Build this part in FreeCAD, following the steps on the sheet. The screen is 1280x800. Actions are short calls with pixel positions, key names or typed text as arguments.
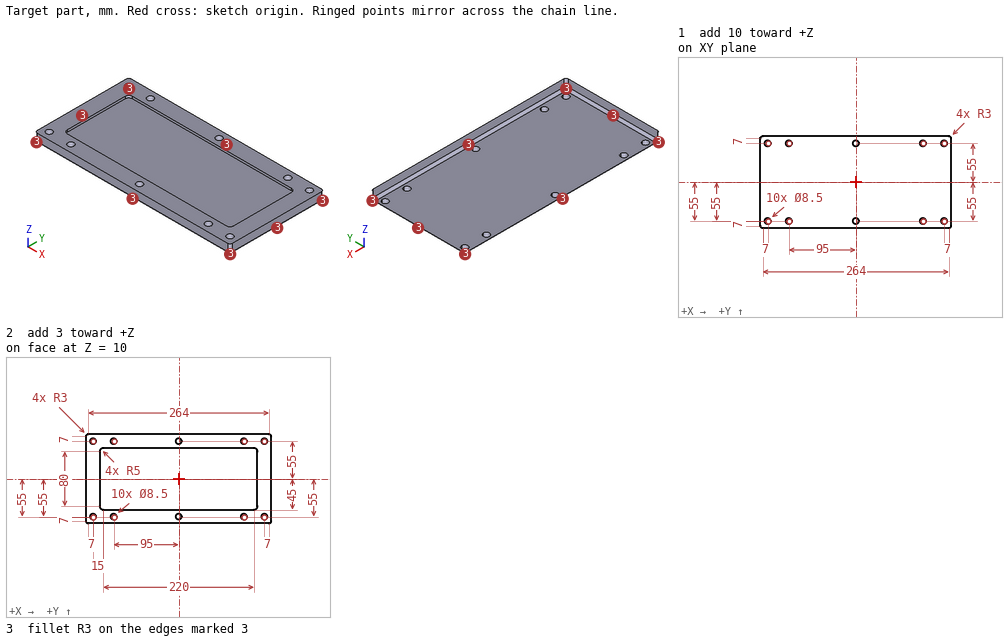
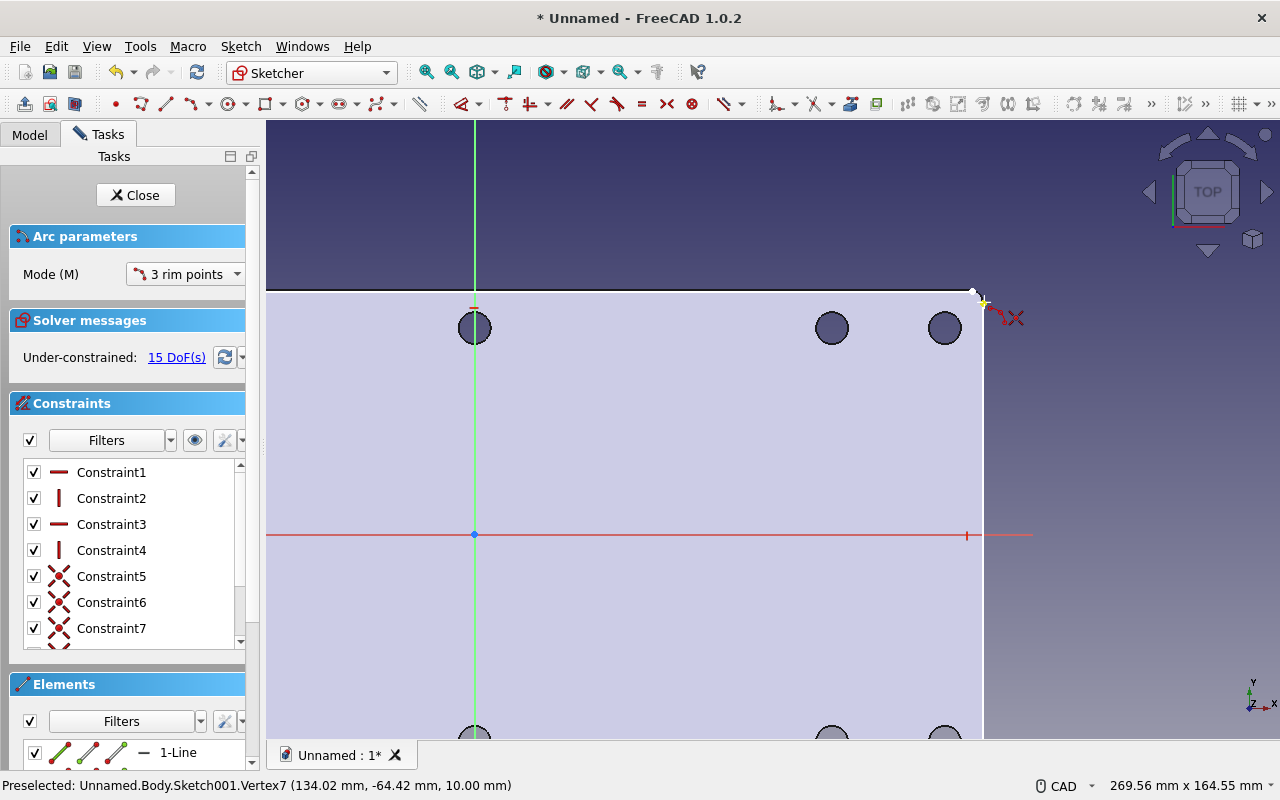
click(983, 303)
click(972, 292)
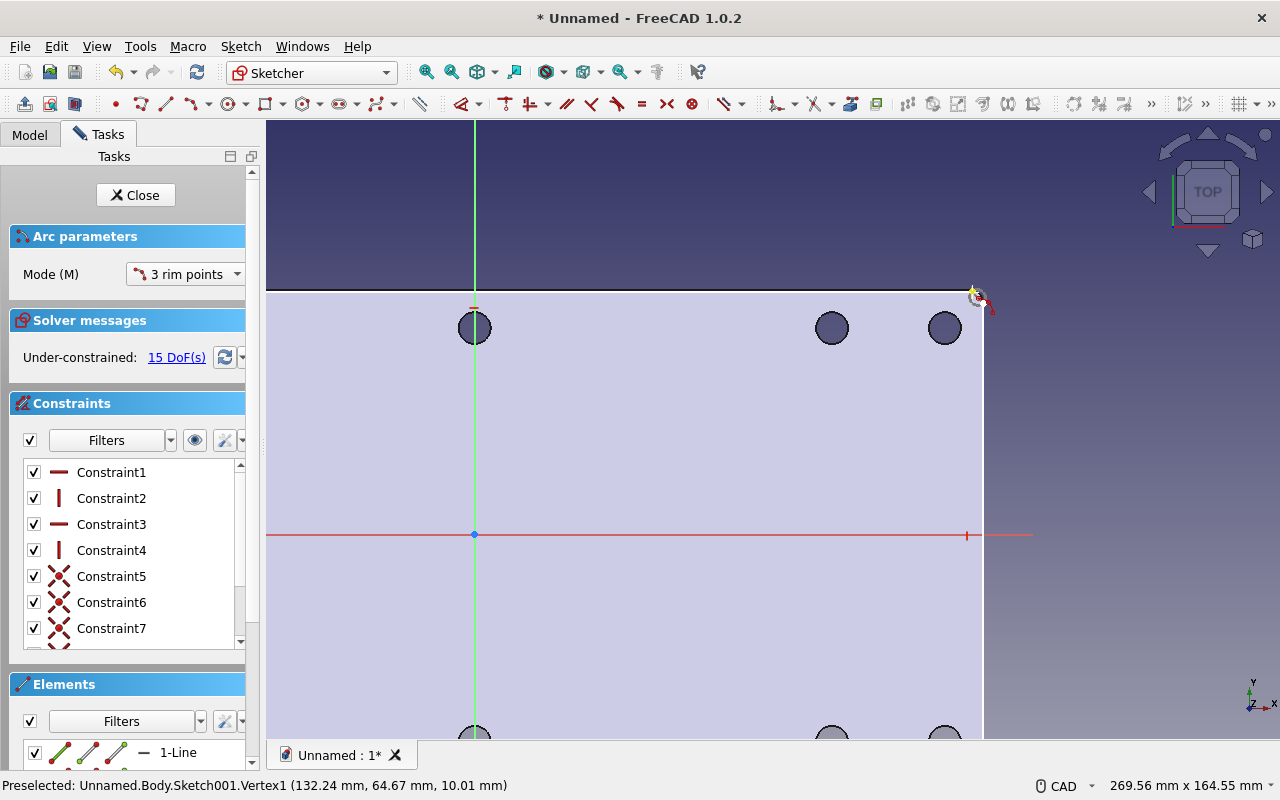
scroll(979, 294, up, 8)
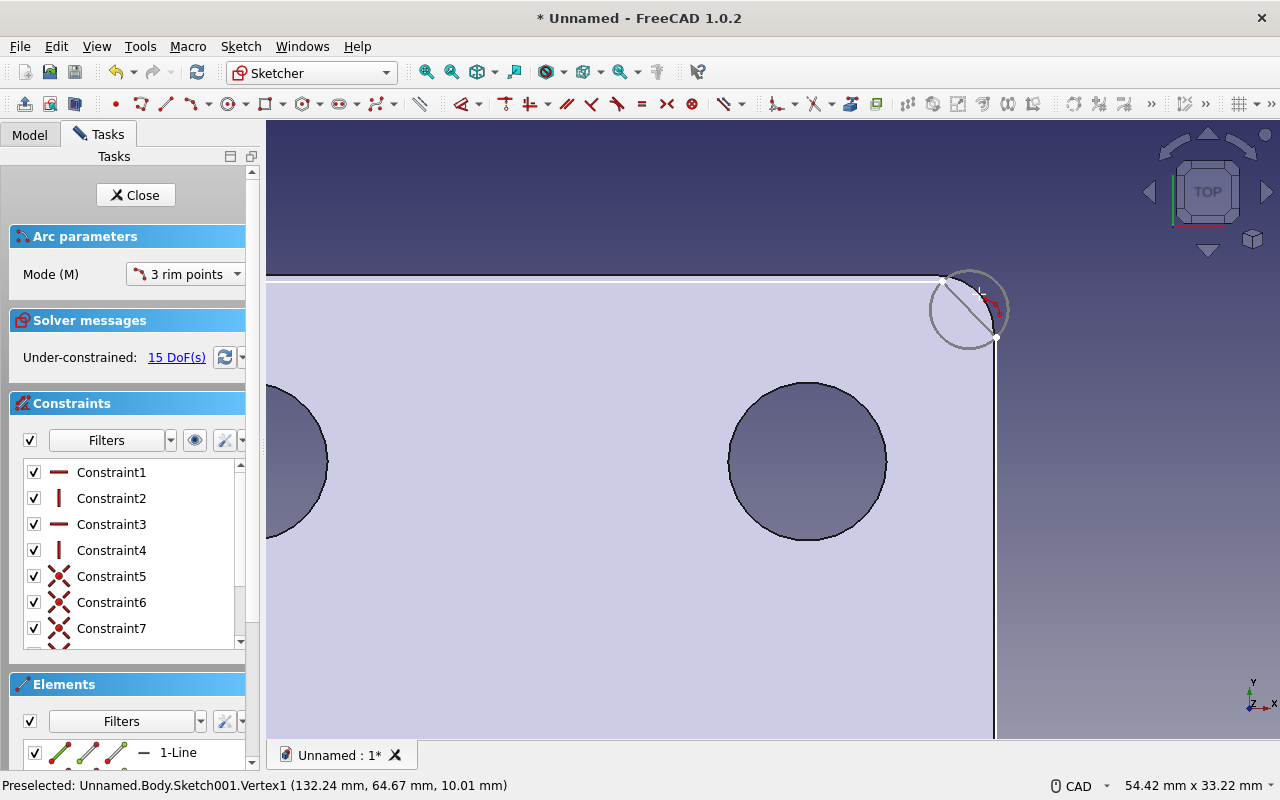
click(977, 292)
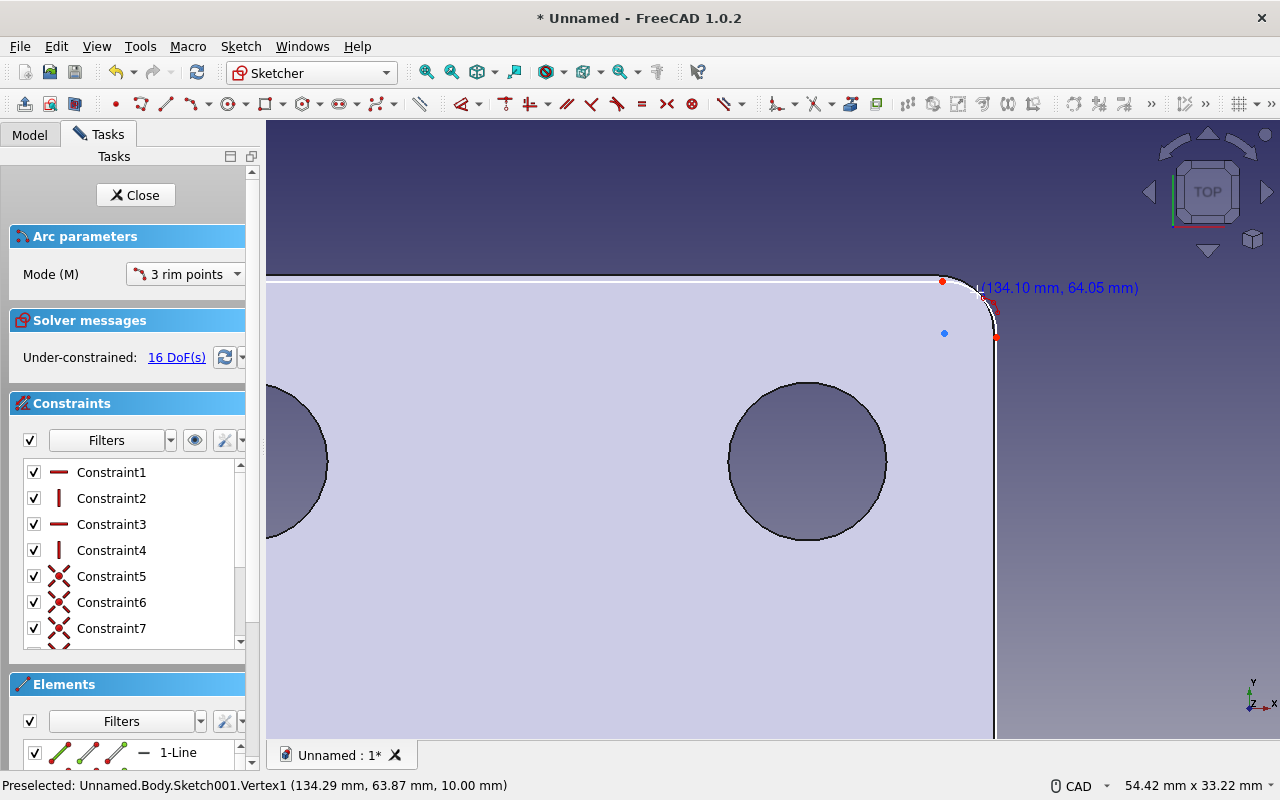
click(166, 104)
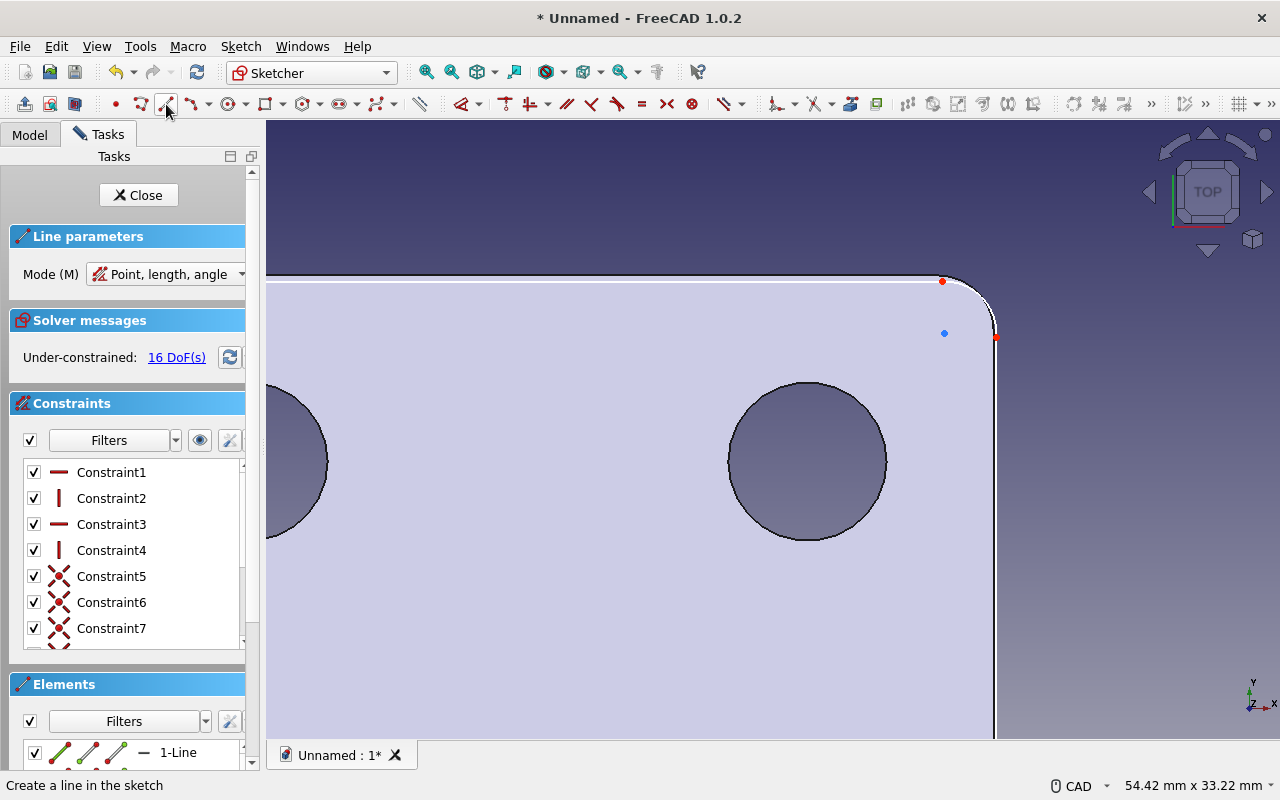
scroll(982, 298, down, 11)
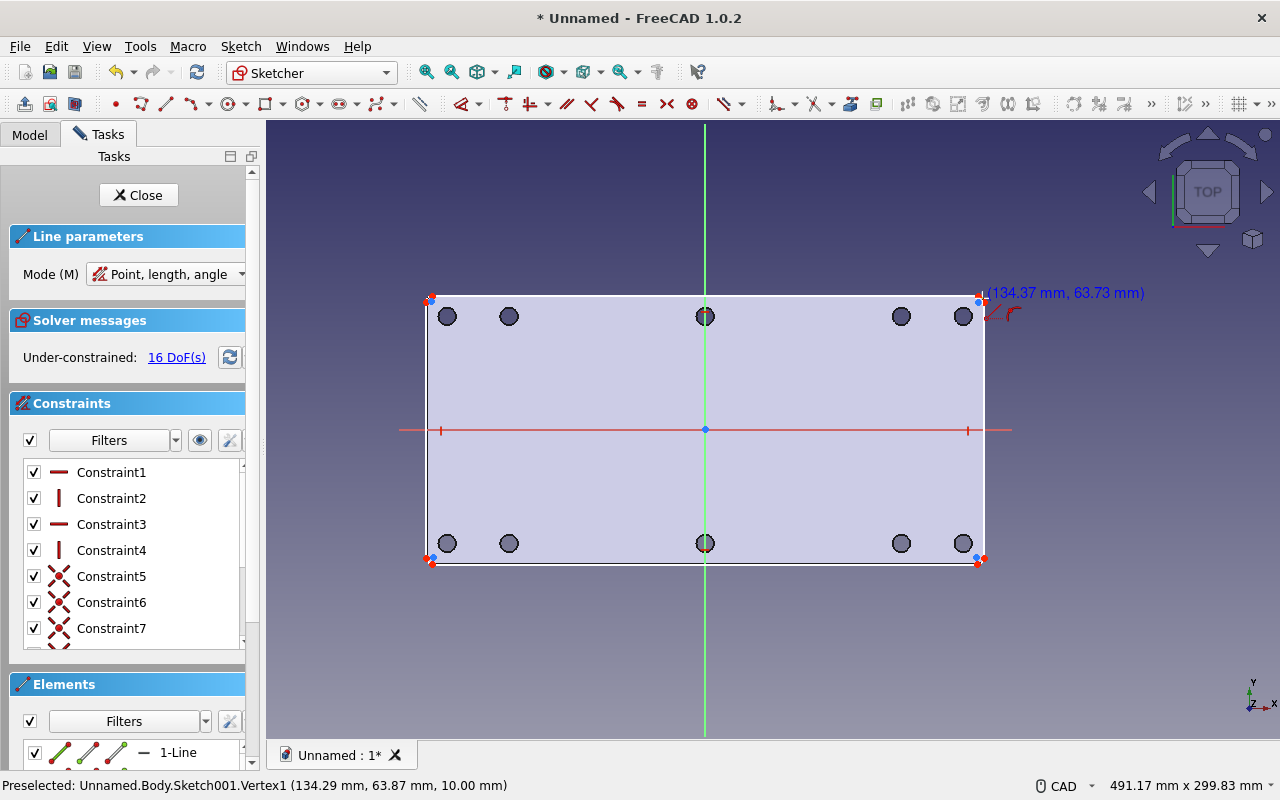
click(932, 523)
click(478, 523)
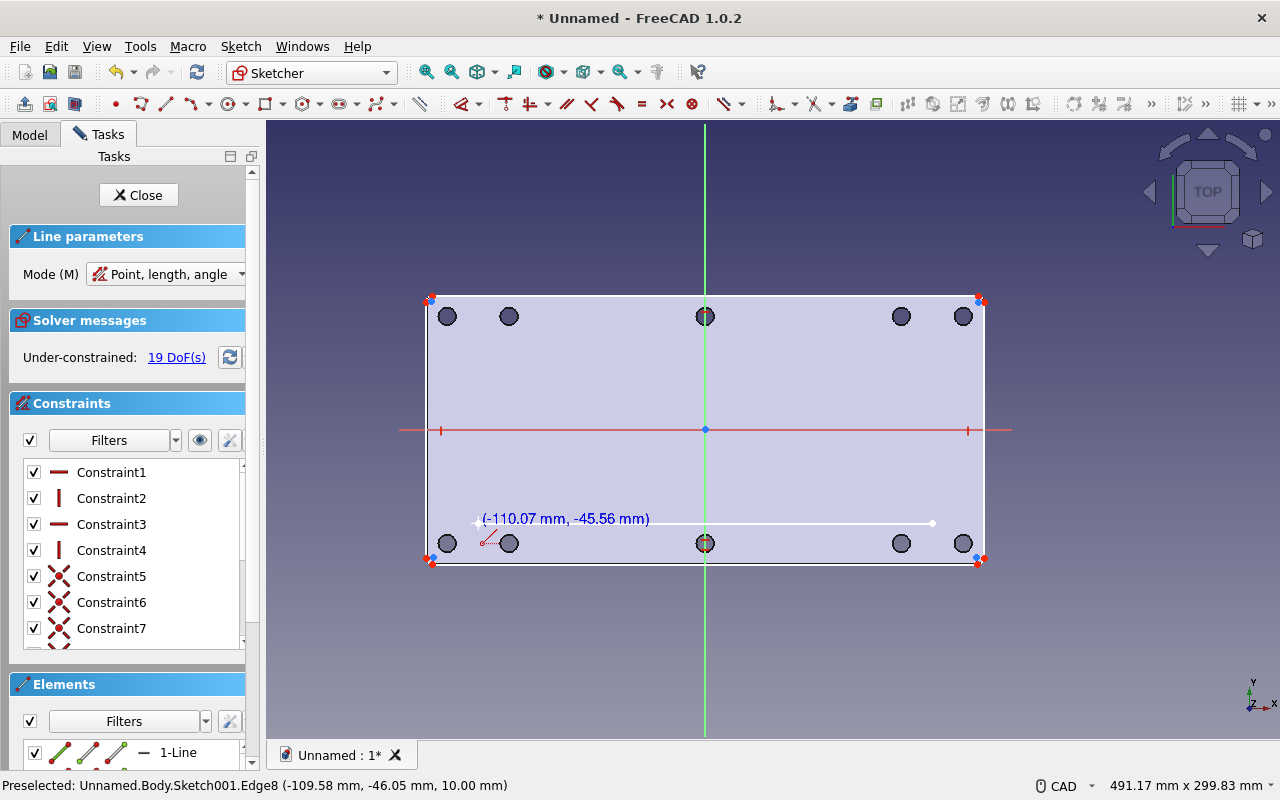
click(468, 513)
click(468, 347)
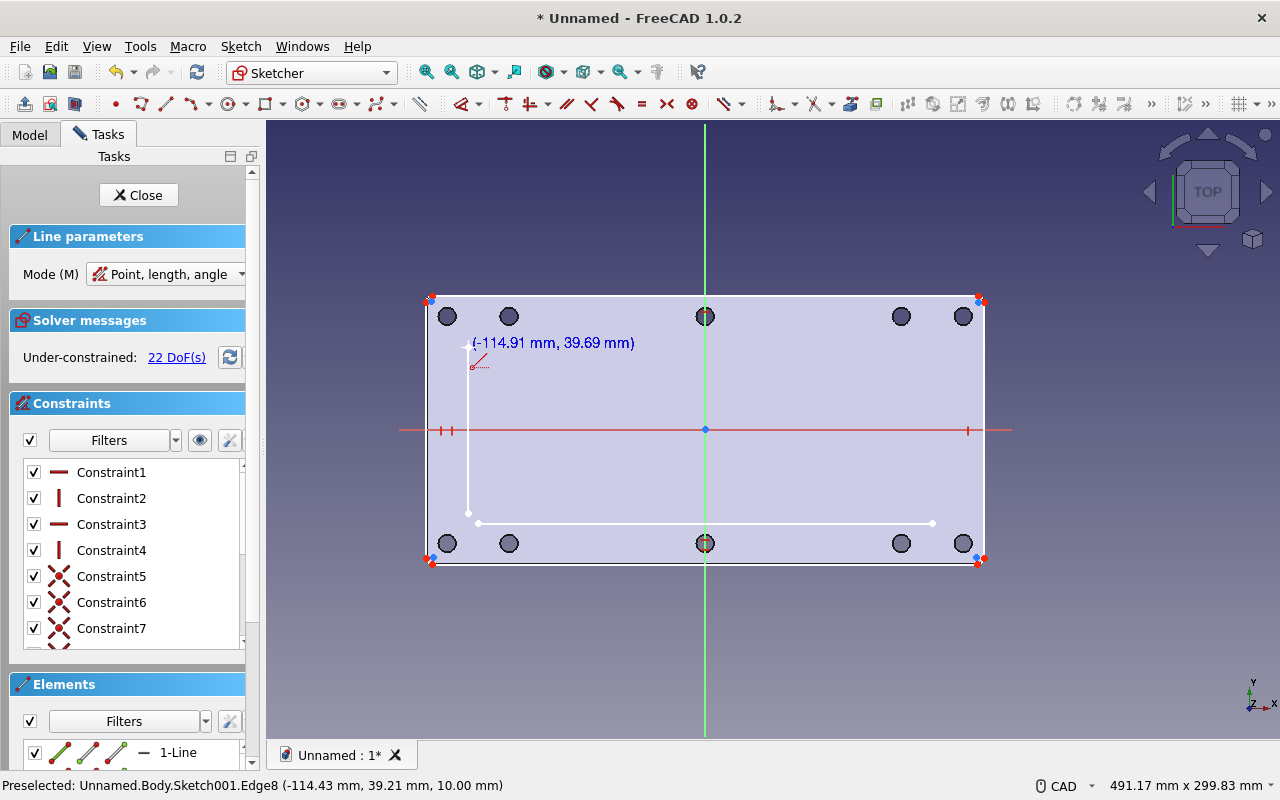
click(478, 337)
click(932, 337)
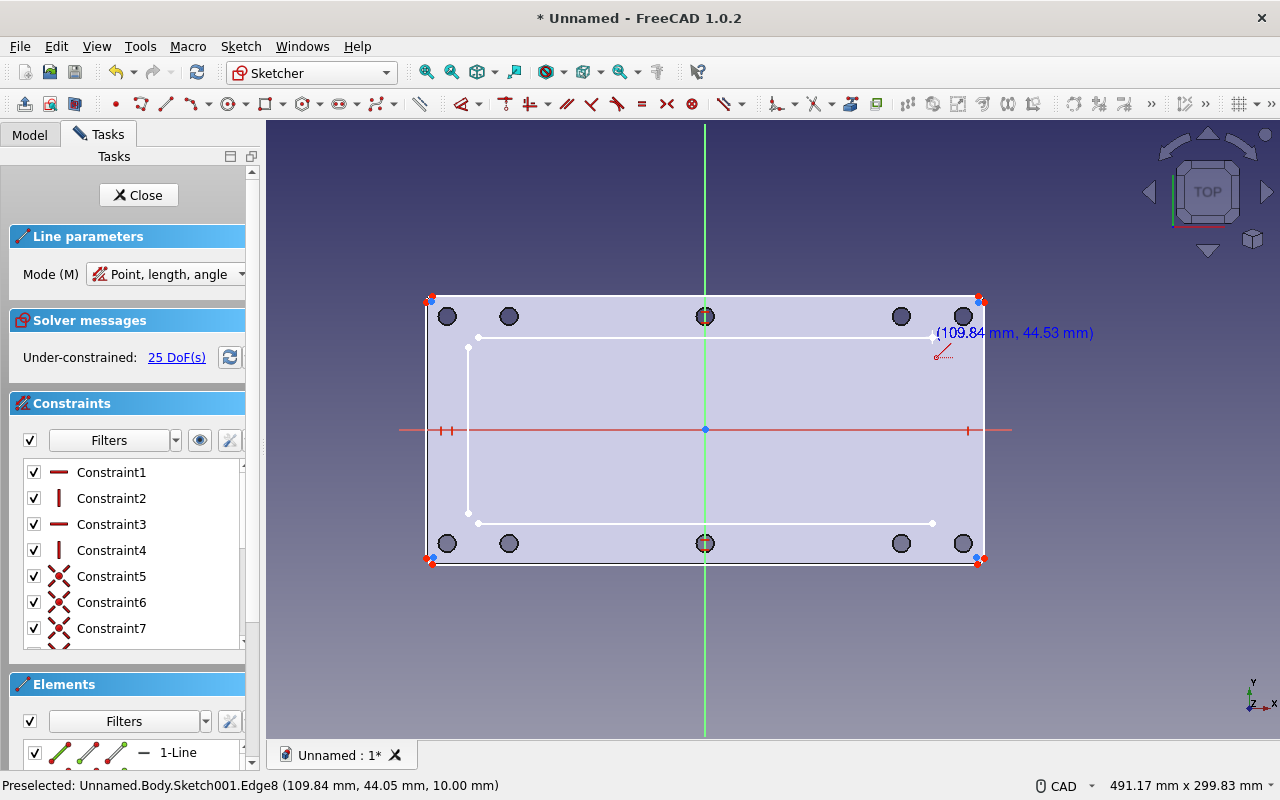
click(943, 347)
click(943, 513)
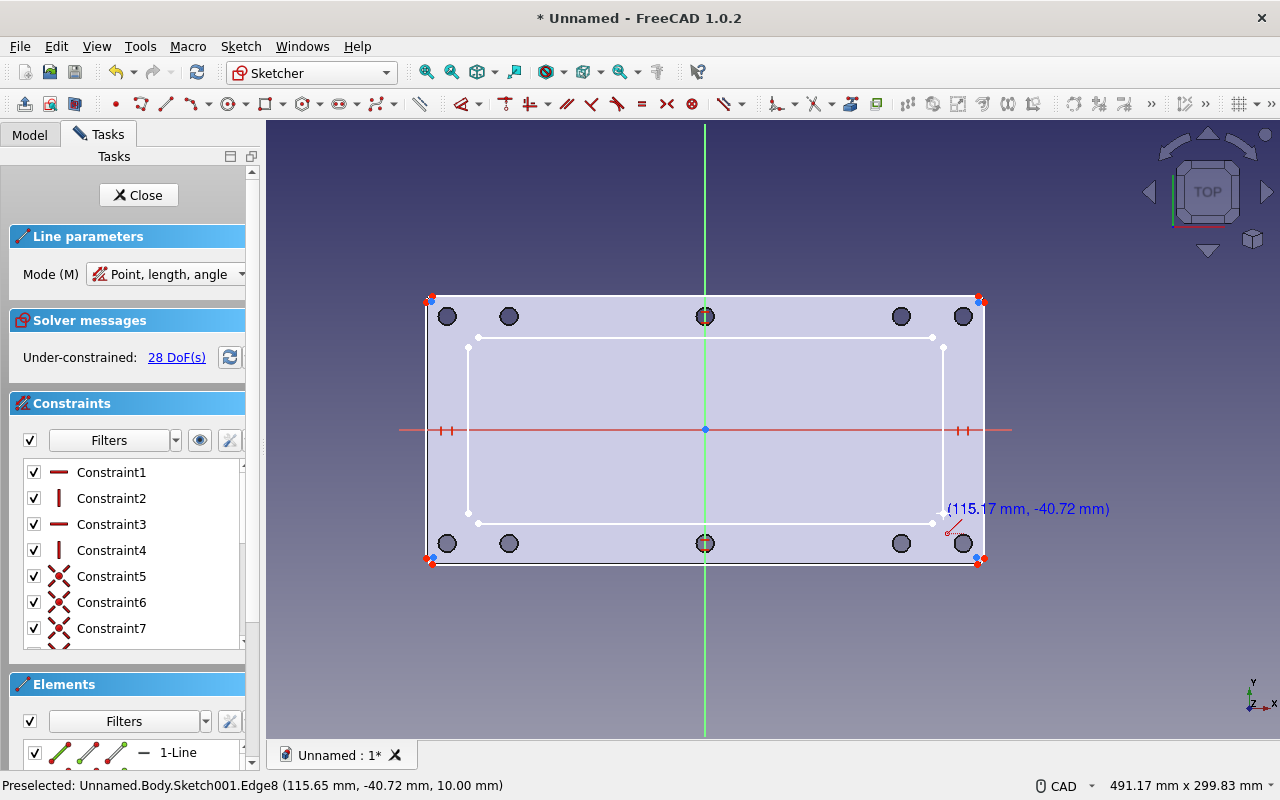
click(190, 104)